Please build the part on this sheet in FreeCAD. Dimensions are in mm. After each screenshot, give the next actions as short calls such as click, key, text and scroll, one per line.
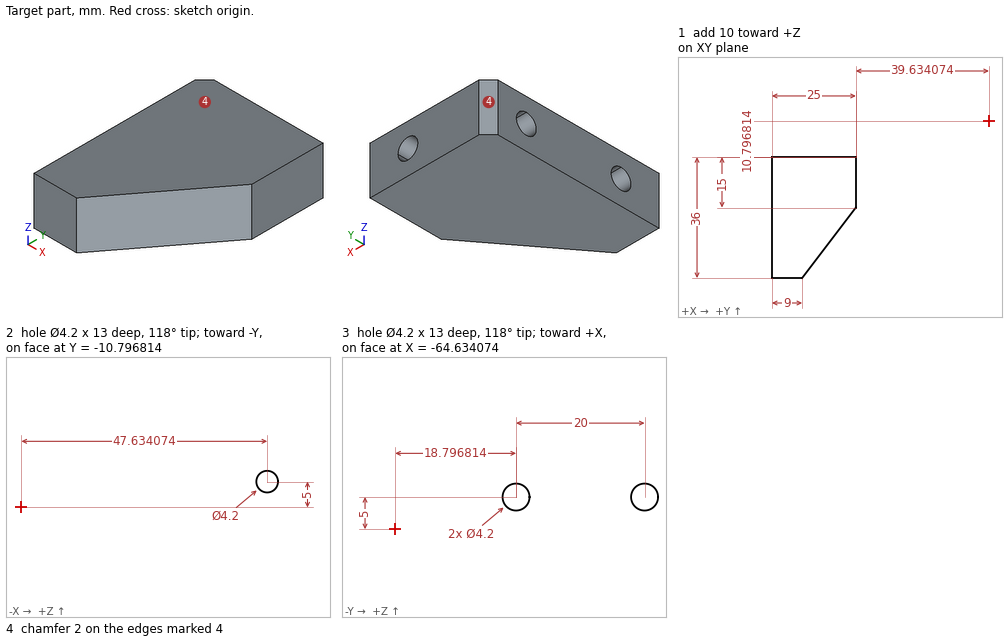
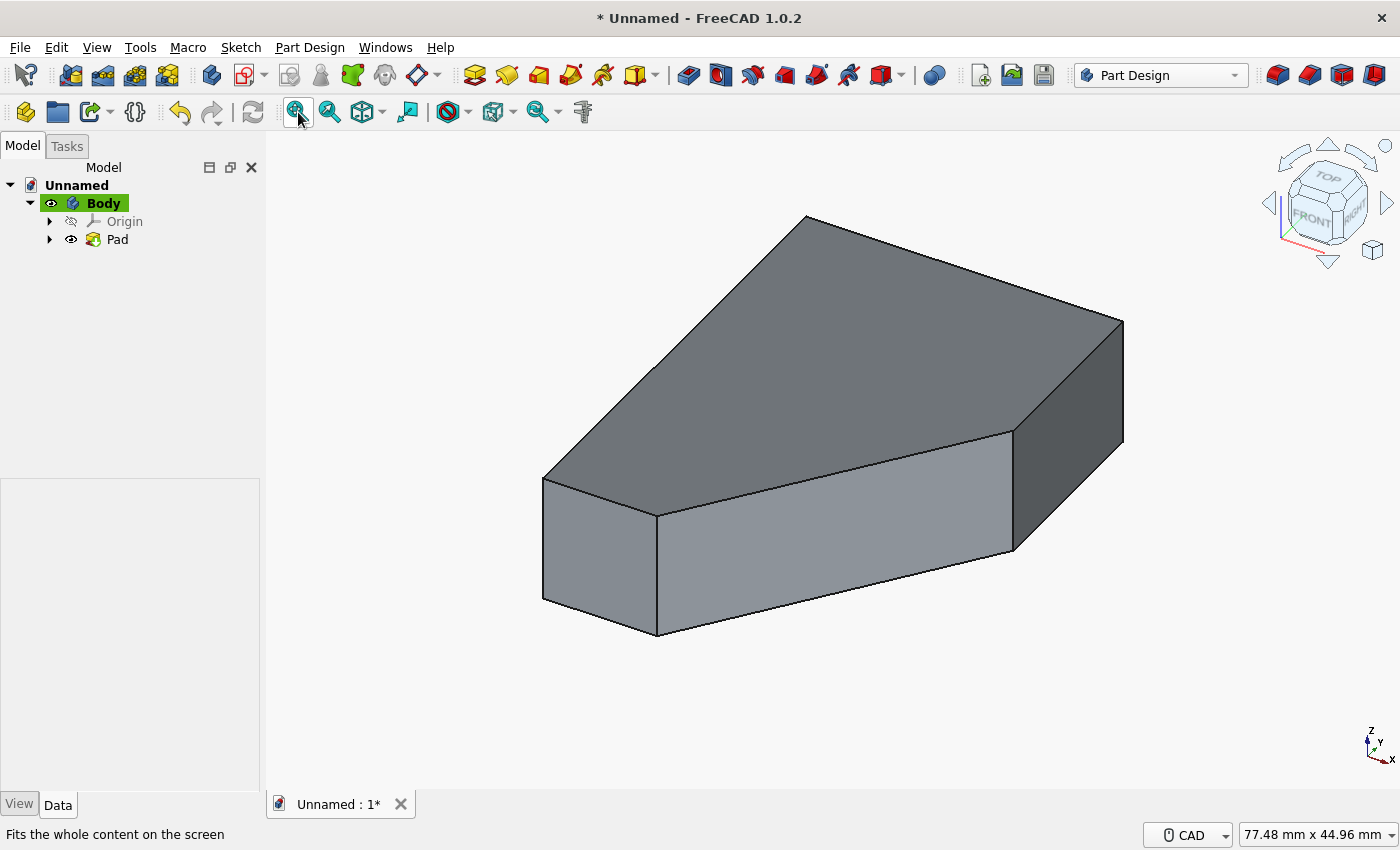
key(4)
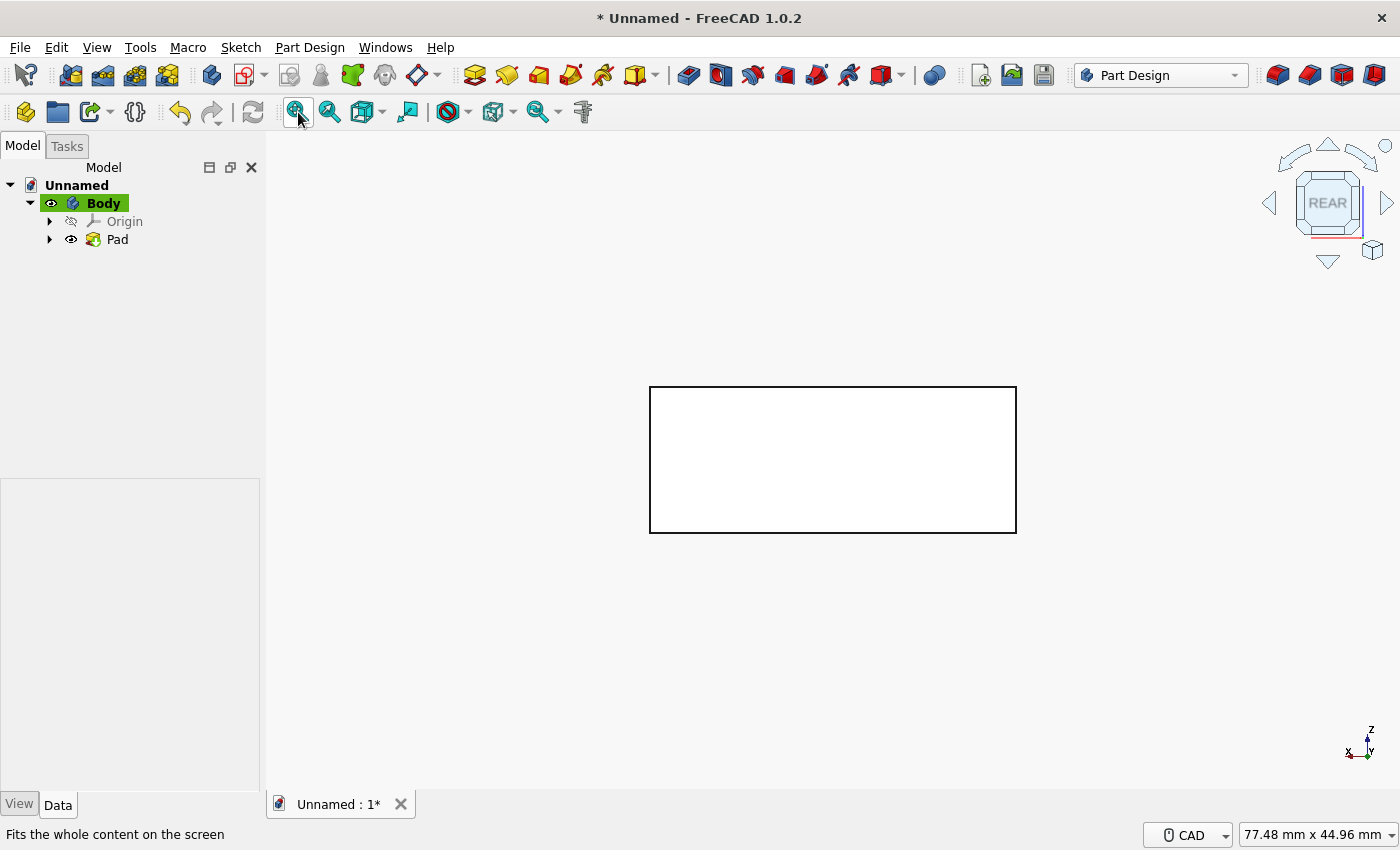
click(298, 112)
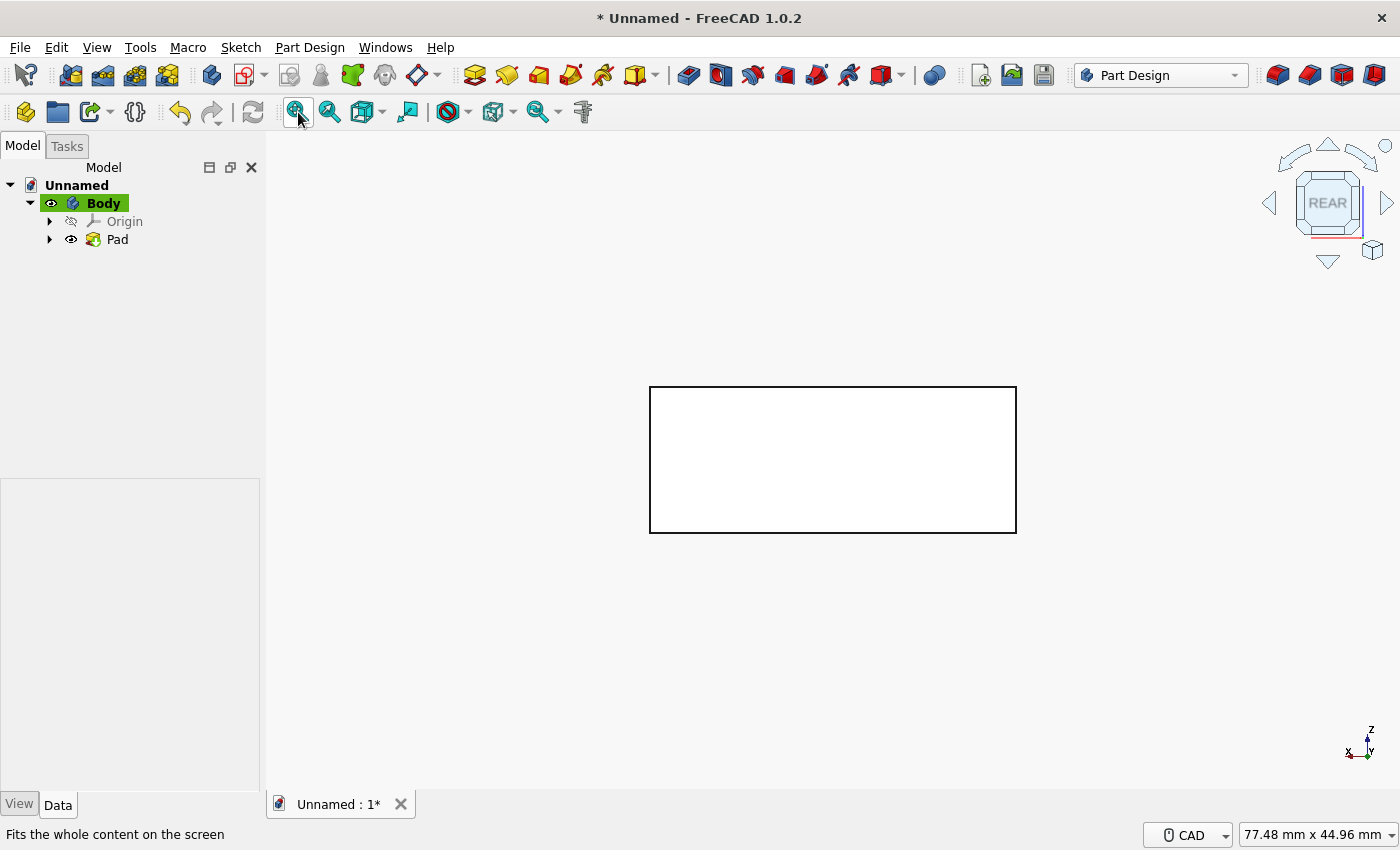
click(728, 459)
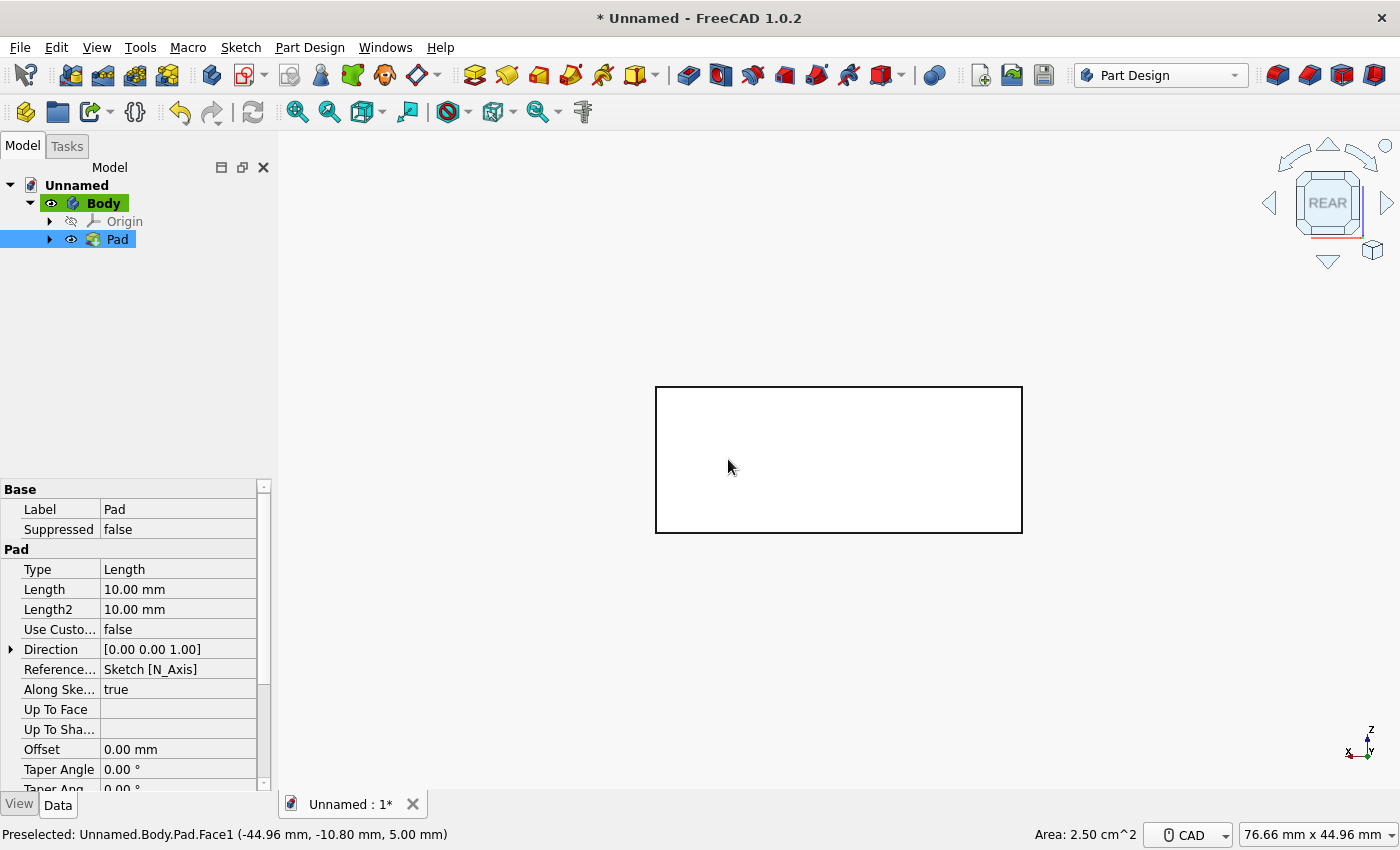
click(244, 76)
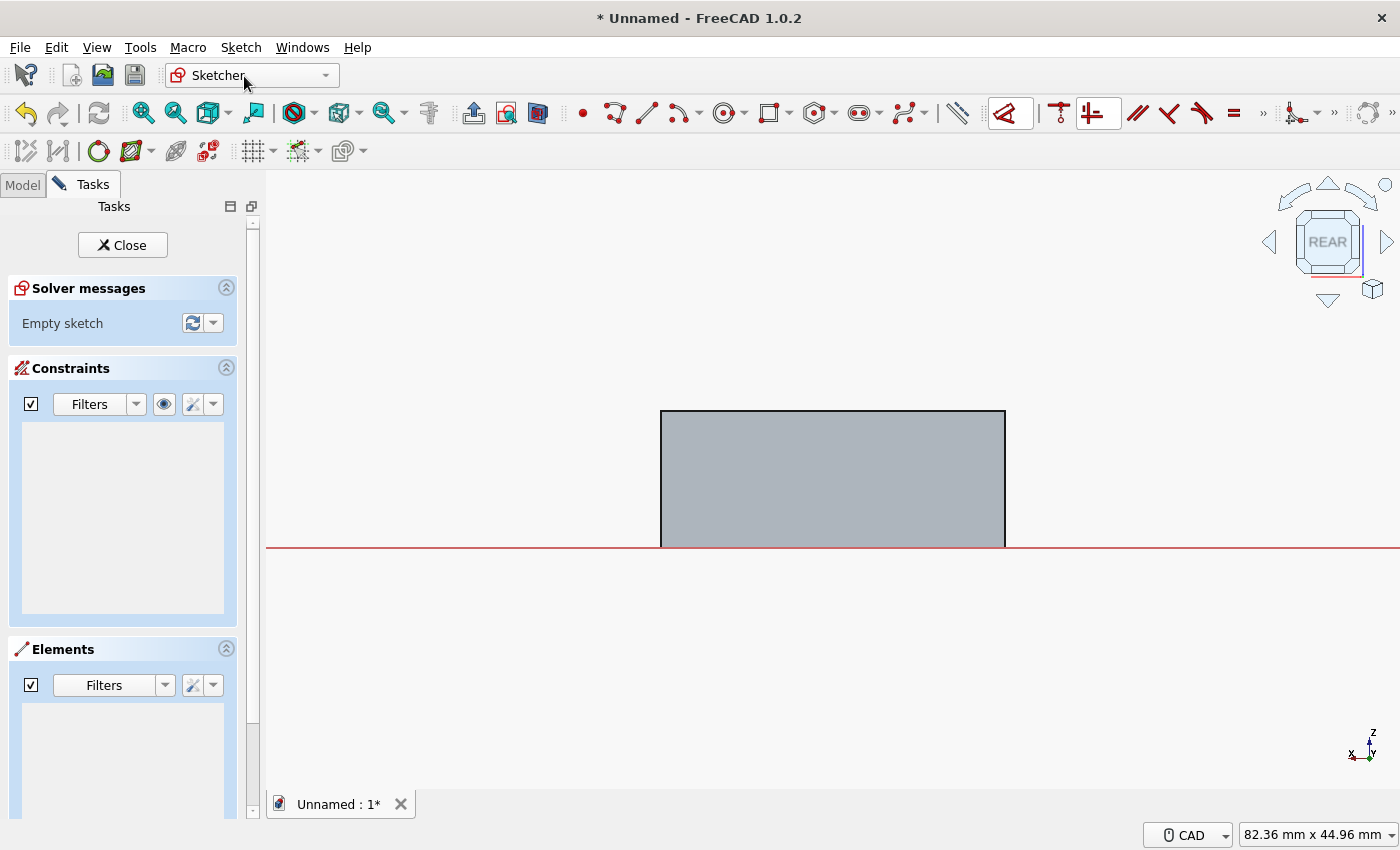
scroll(772, 480, up, 10)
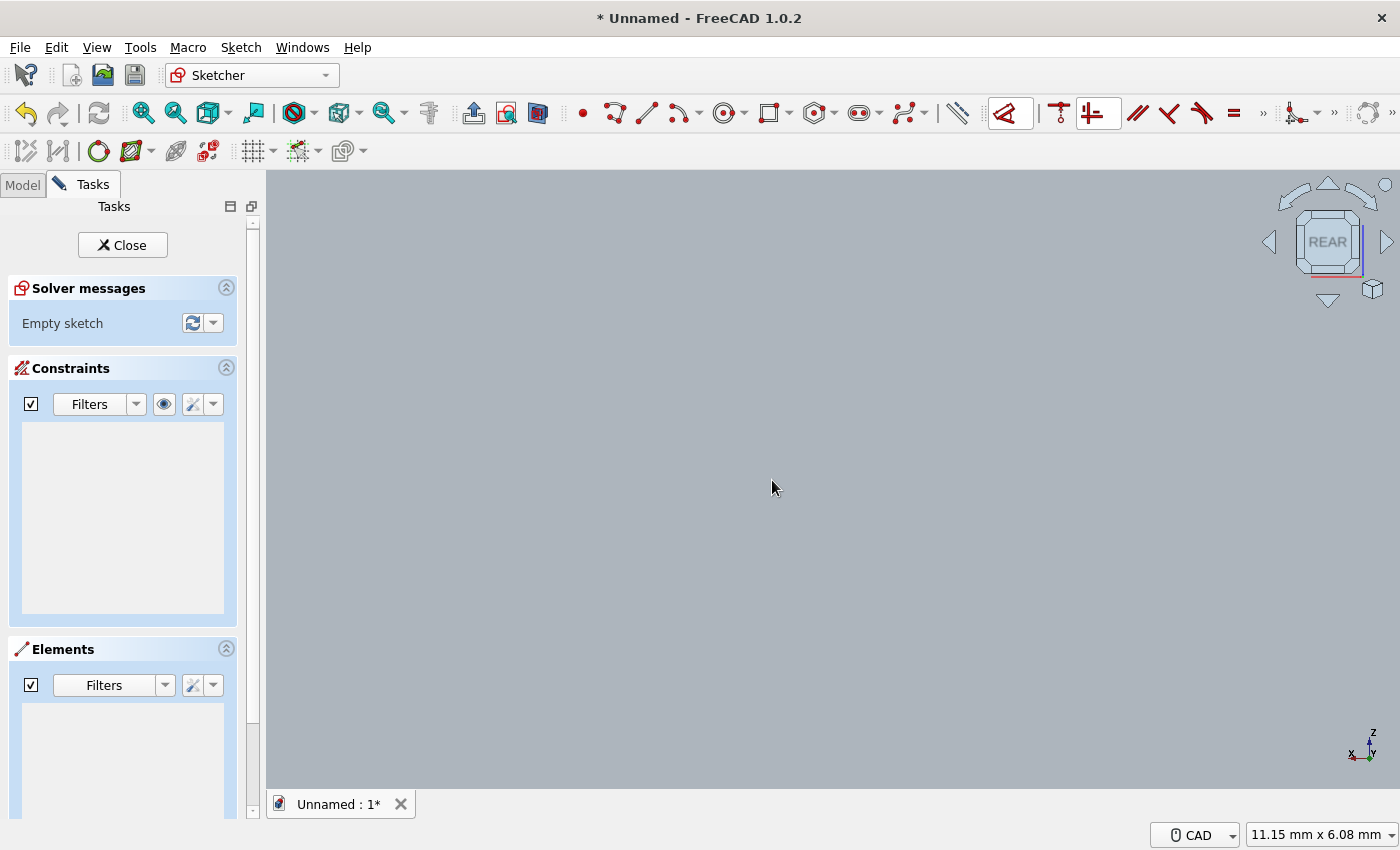
click(724, 114)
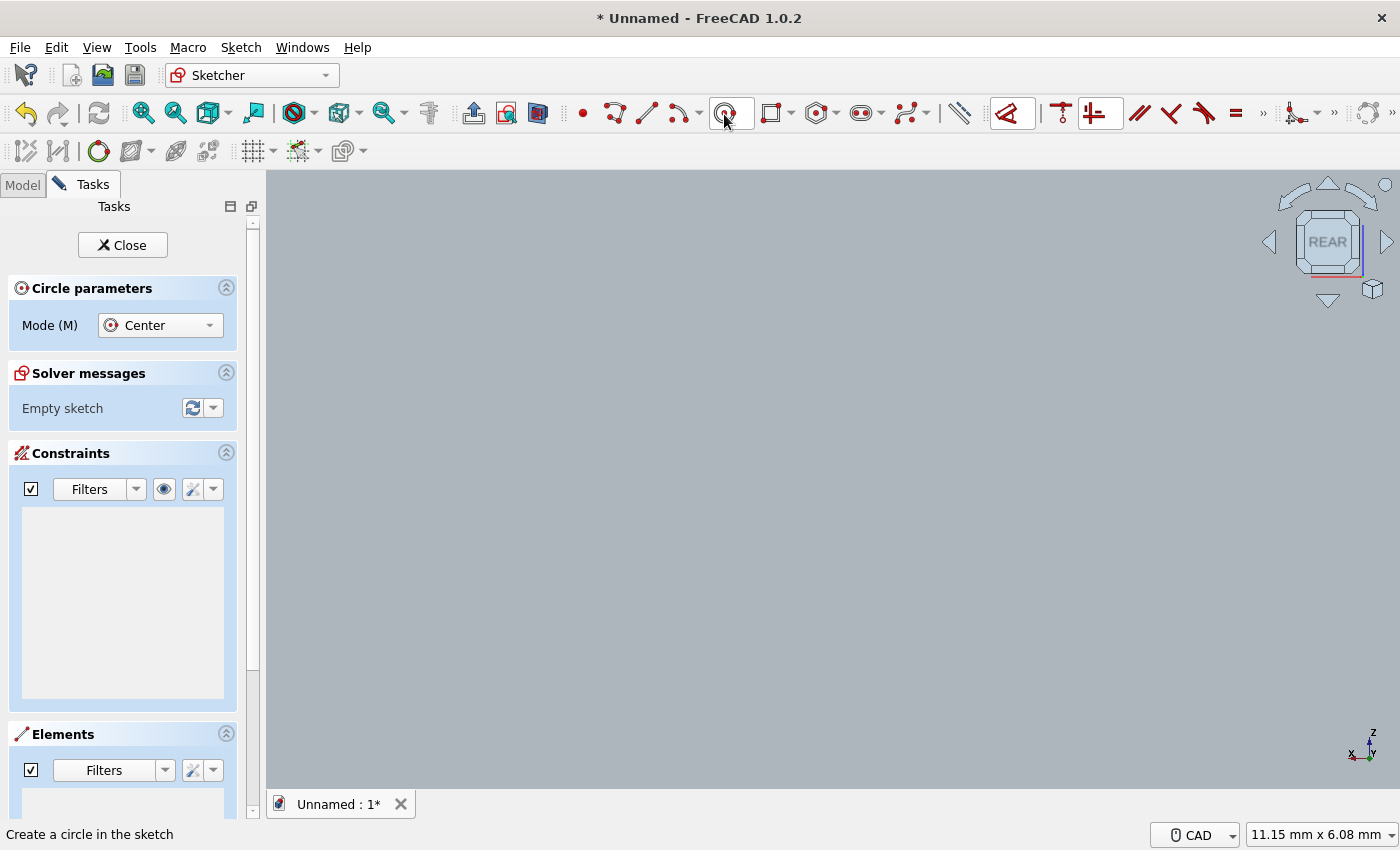
click(762, 473)
move(913, 322)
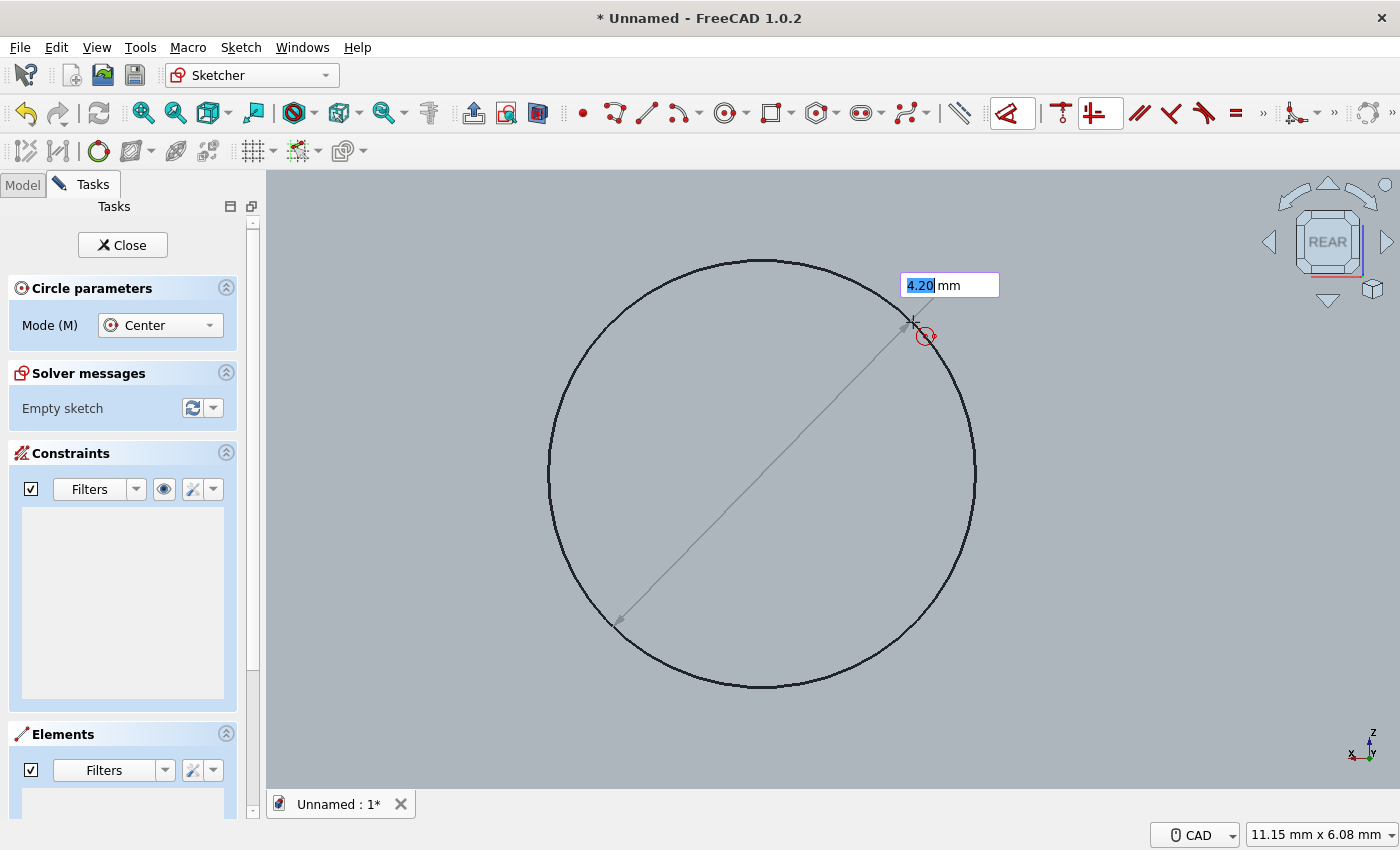
text(4.2)
key(Return)
key(Escape)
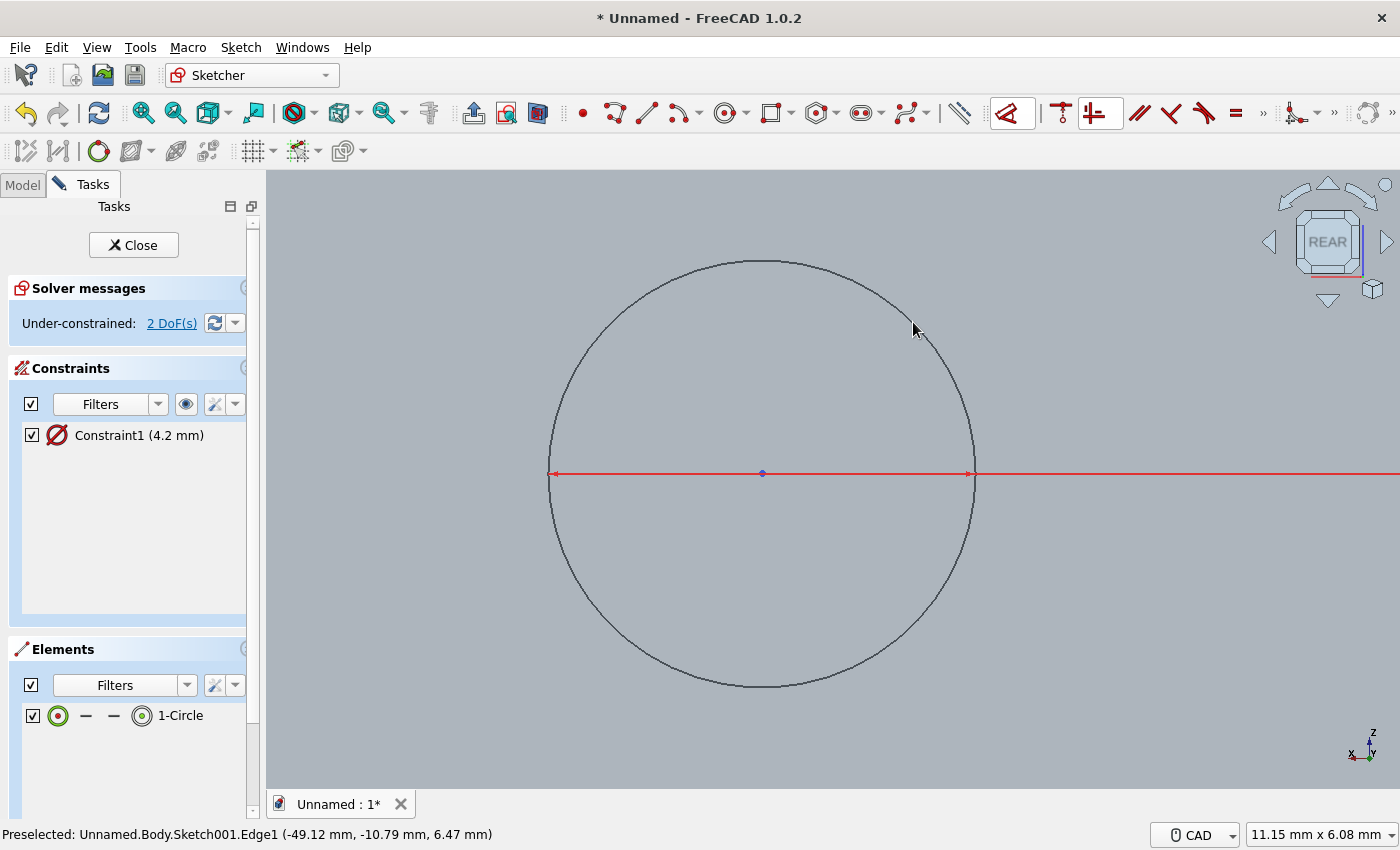
click(762, 474)